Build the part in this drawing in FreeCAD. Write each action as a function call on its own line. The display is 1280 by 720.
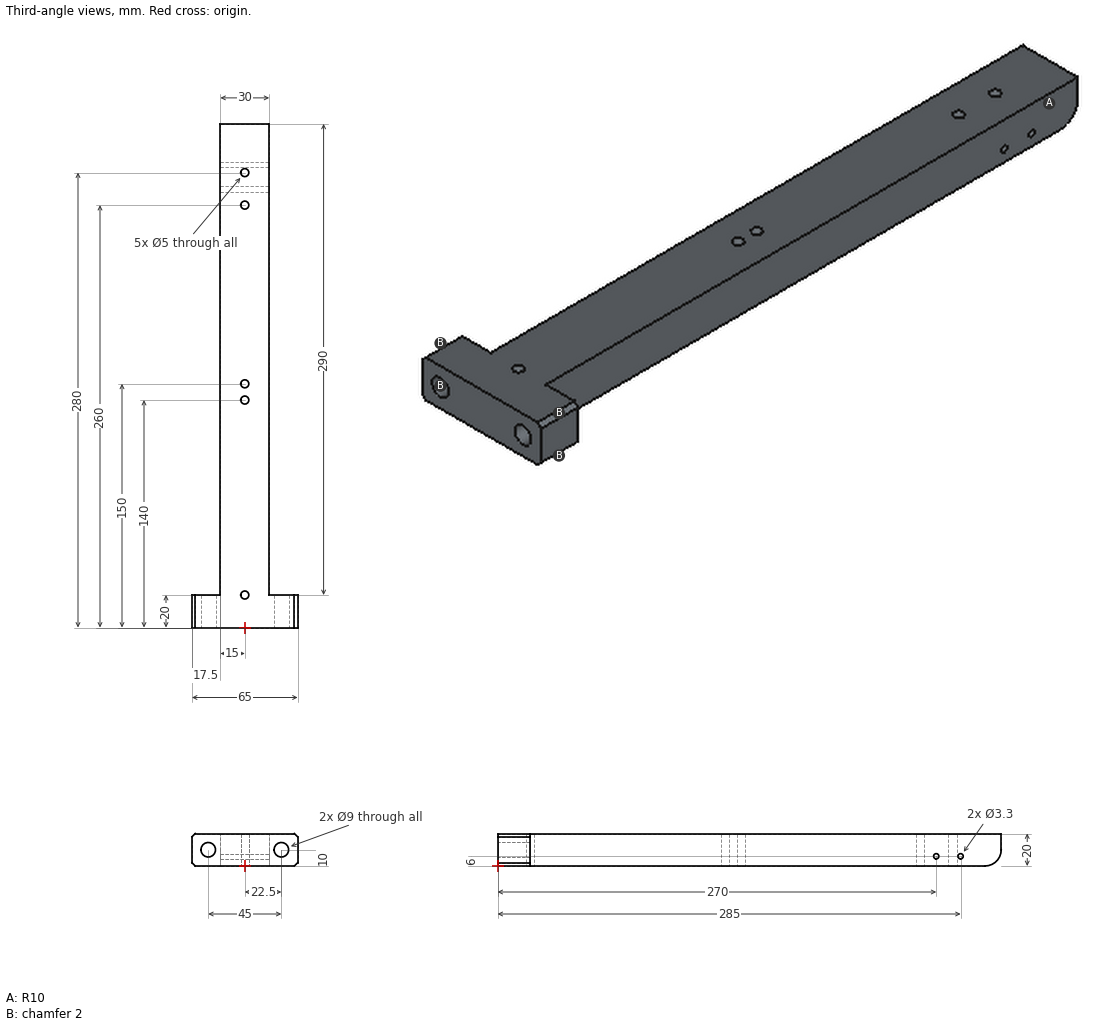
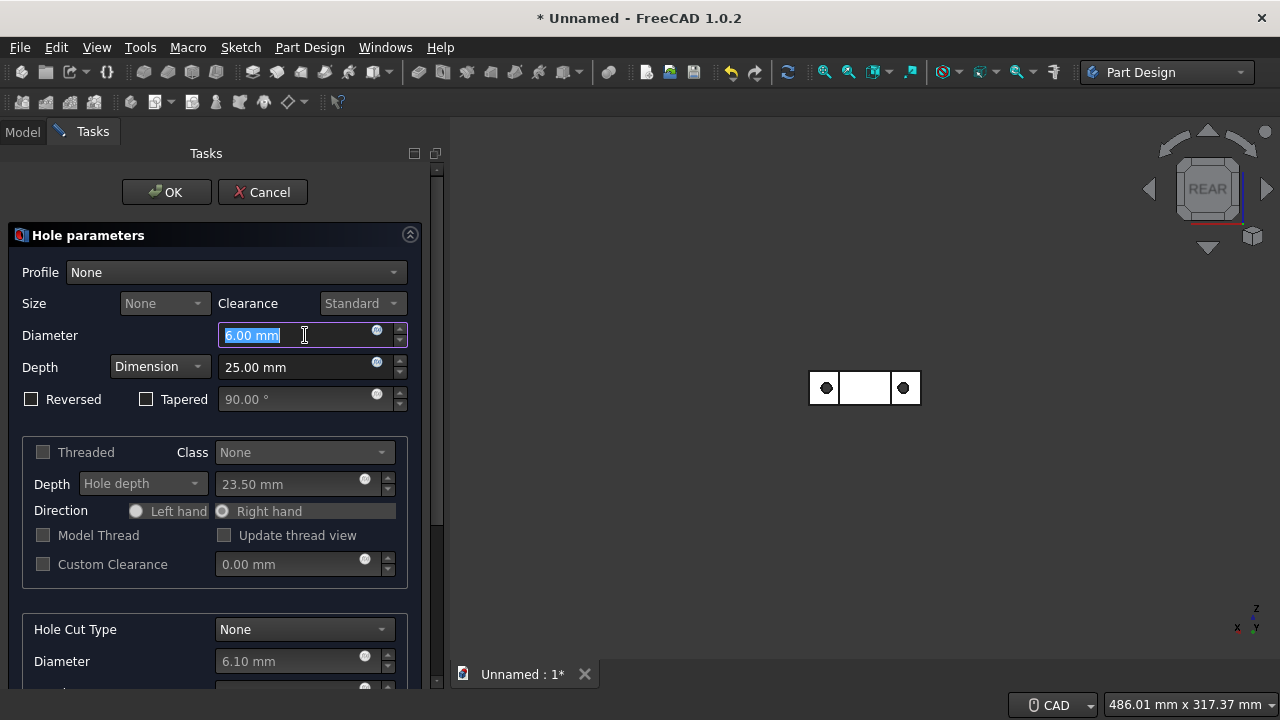
text(9)
key(Tab)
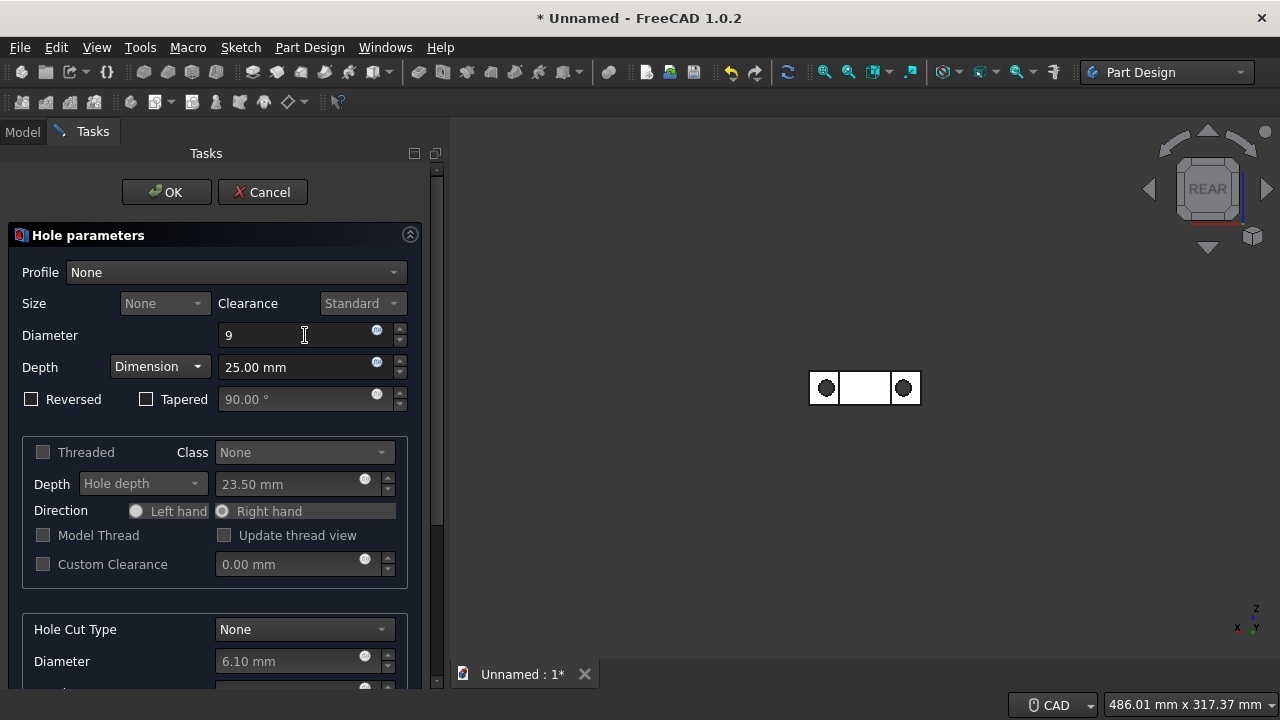
click(161, 366)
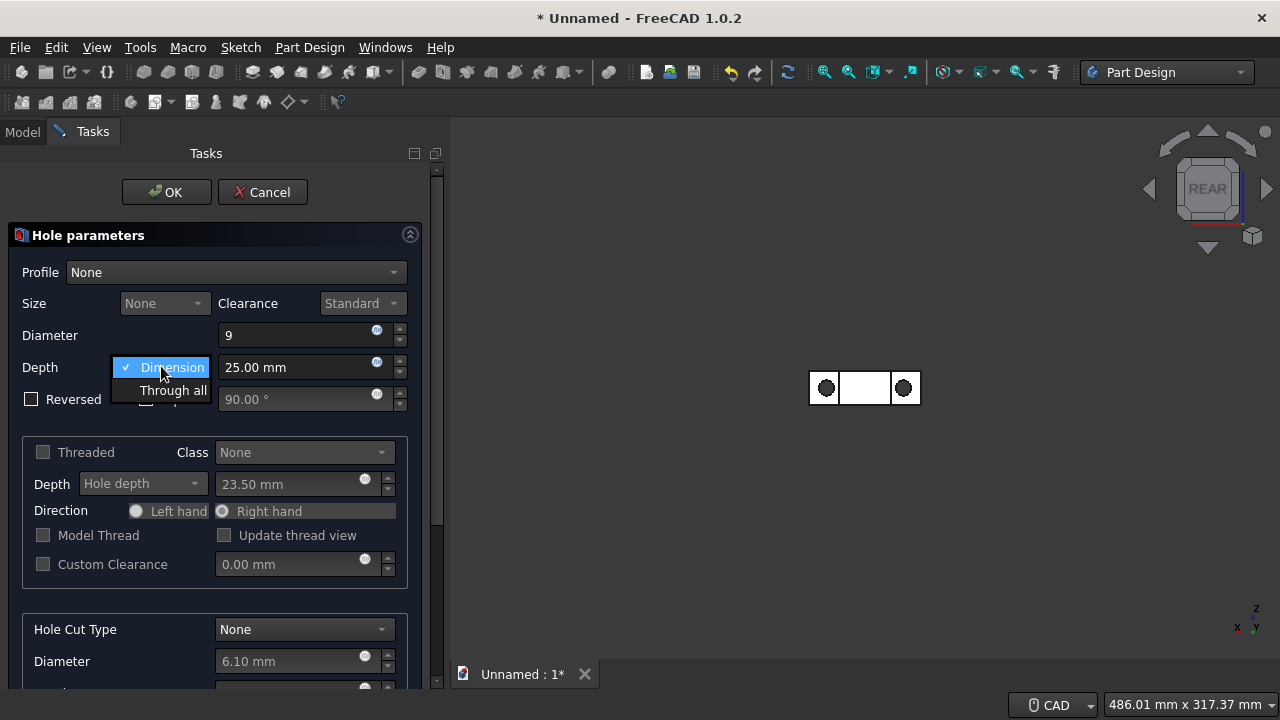
click(160, 390)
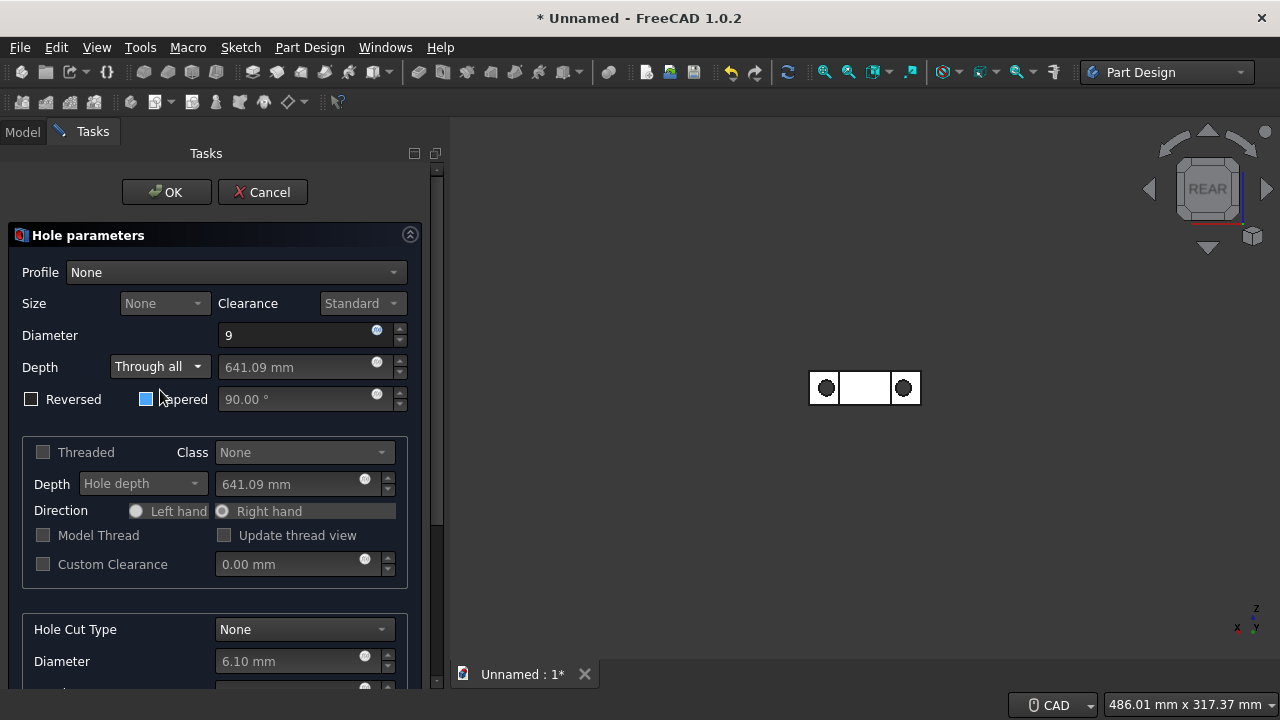
click(167, 192)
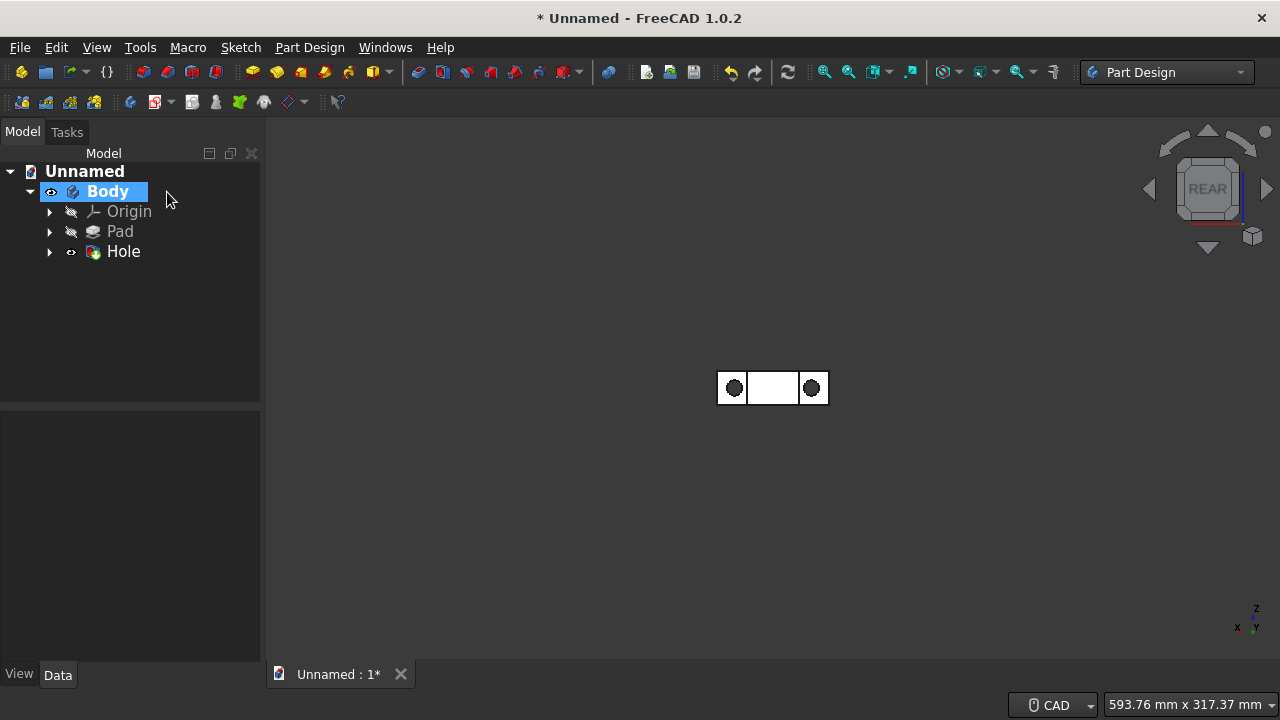
key(v)
key(f)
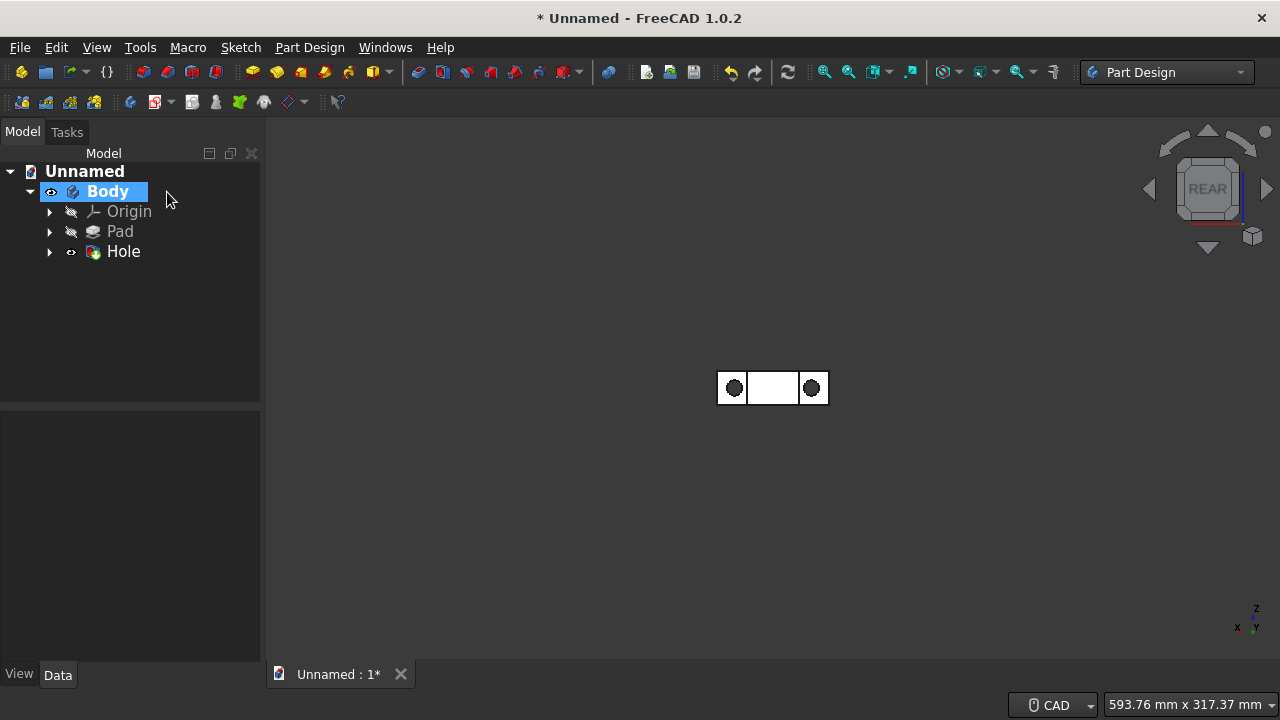
key(0)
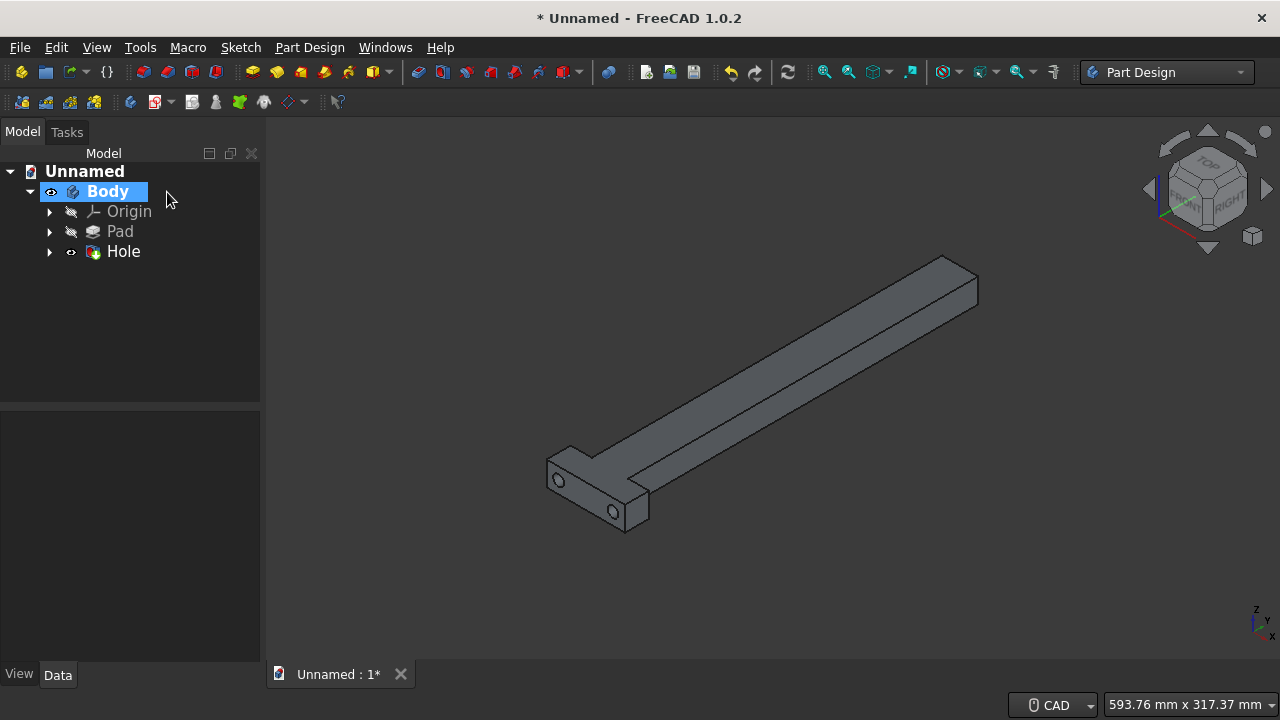
click(933, 280)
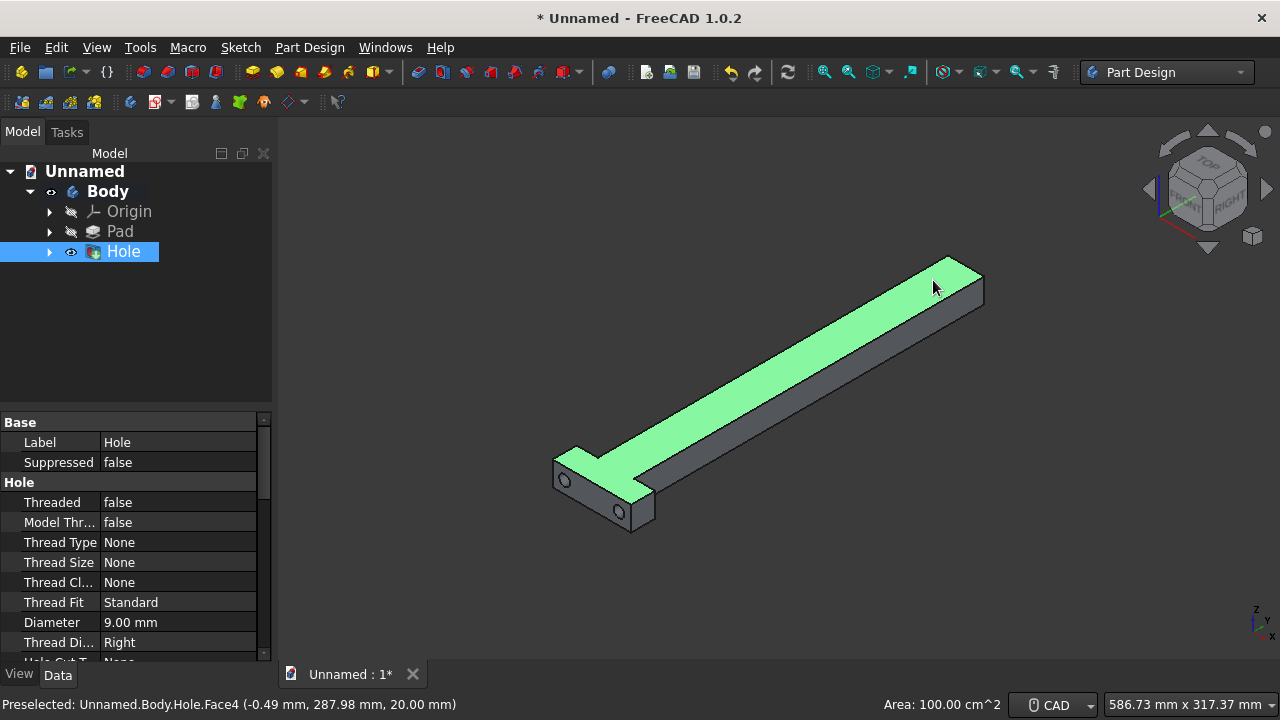
click(156, 102)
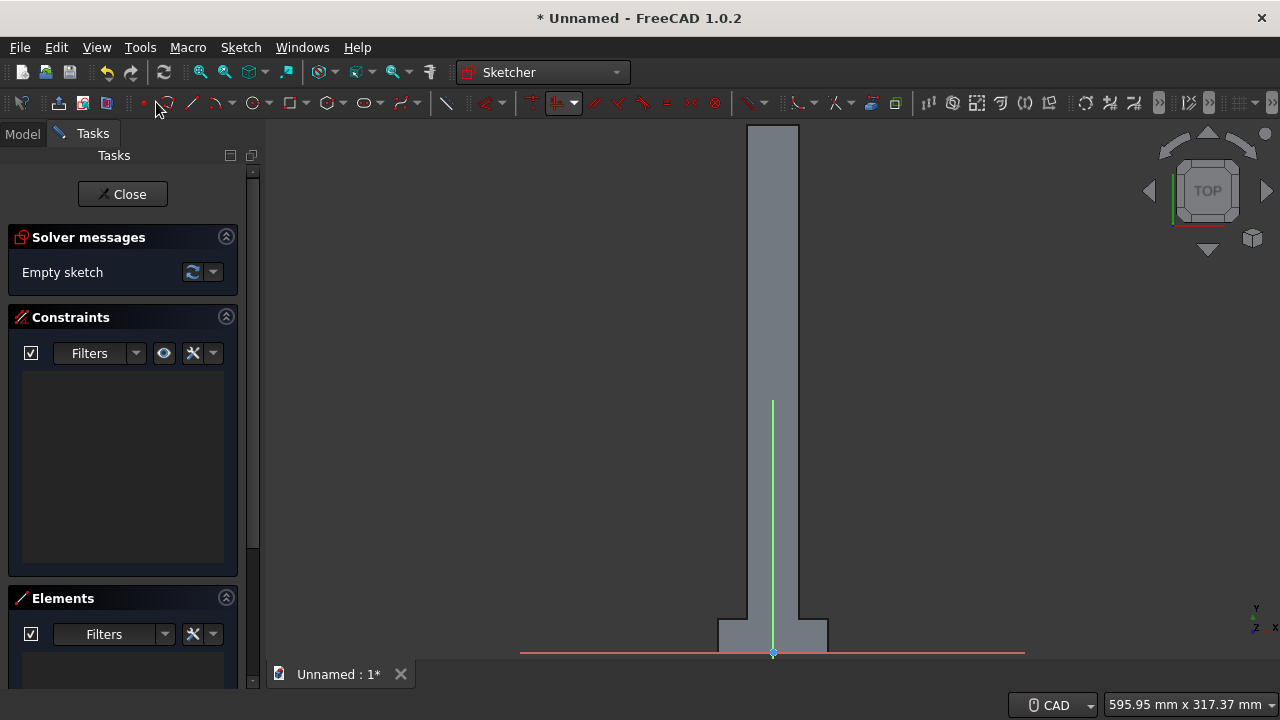
scroll(565, 341, down, 2)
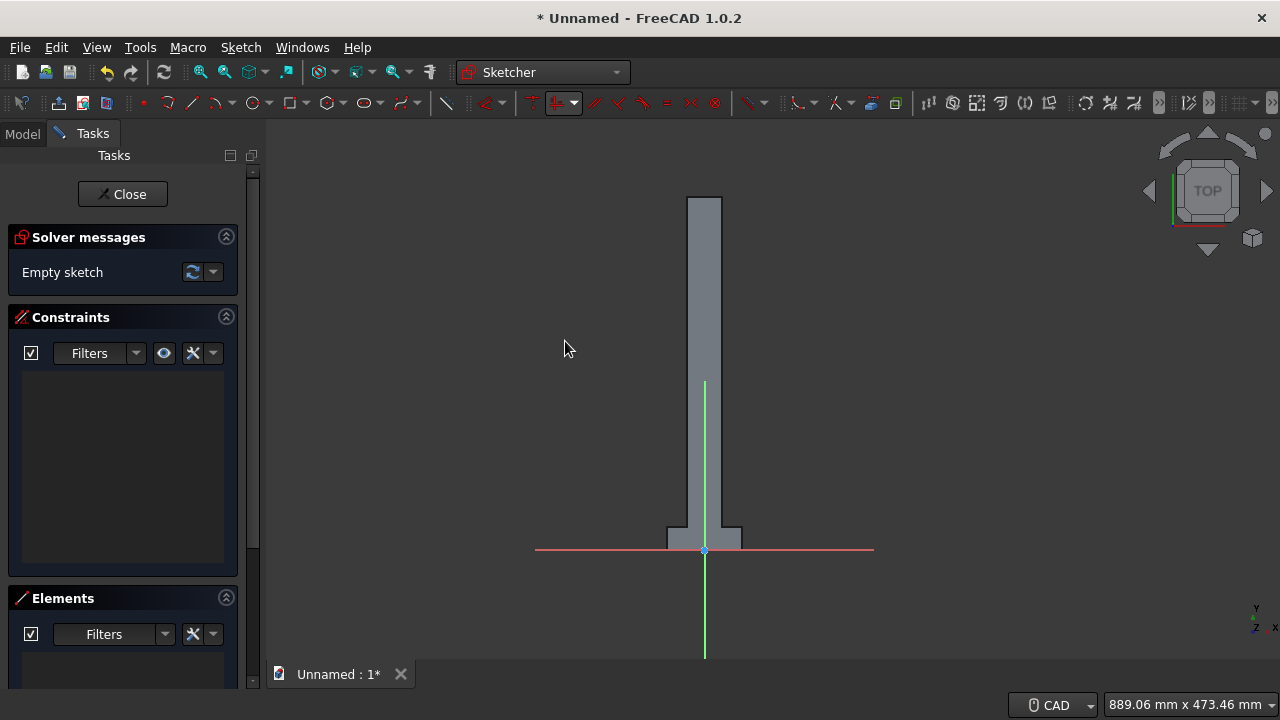
click(254, 104)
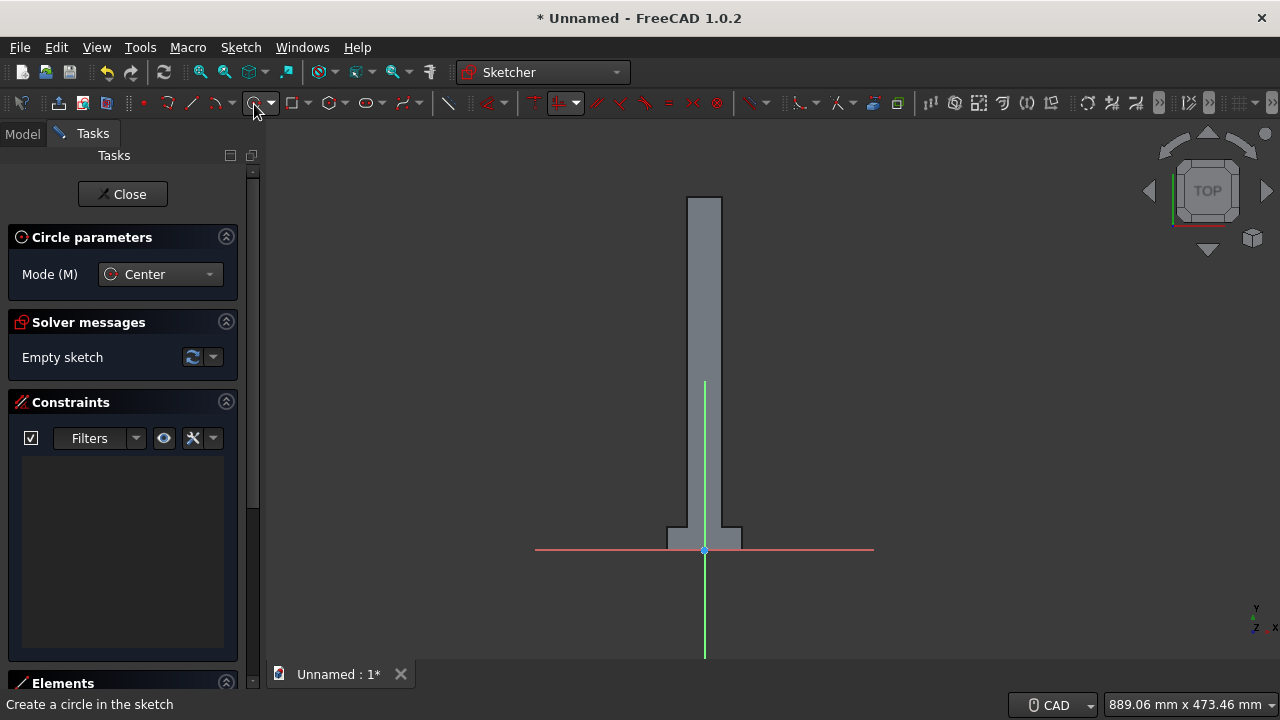
scroll(705, 231, up, 11)